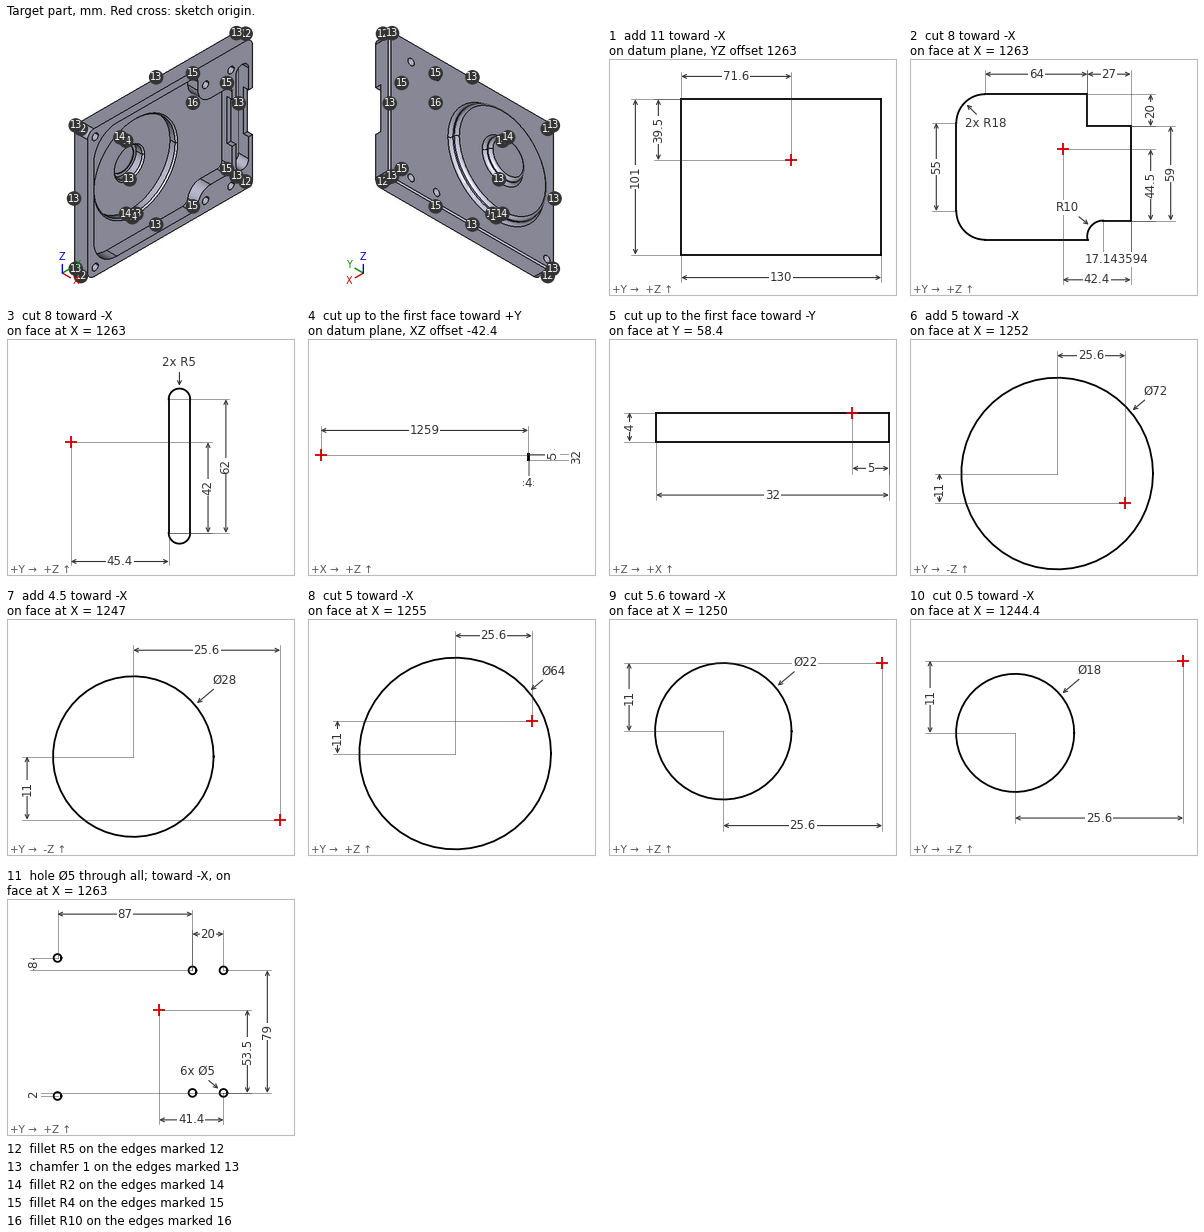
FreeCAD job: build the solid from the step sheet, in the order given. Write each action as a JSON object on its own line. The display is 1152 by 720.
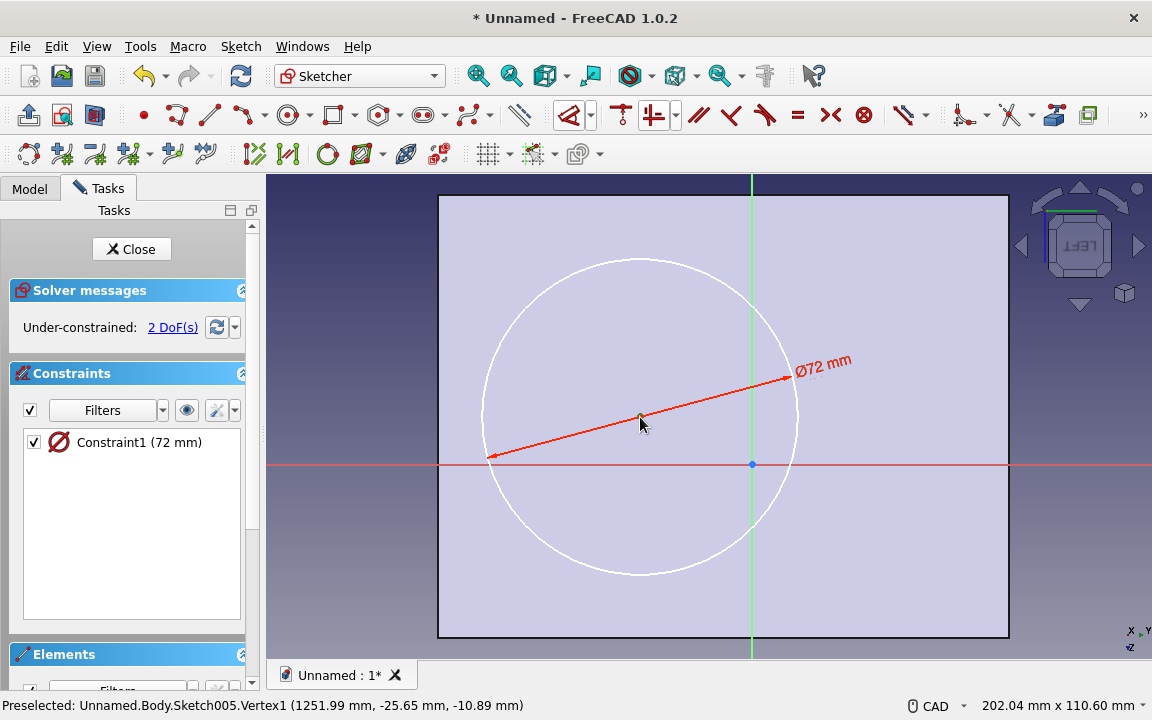
{"action": "left_click", "coordinate": [590, 116]}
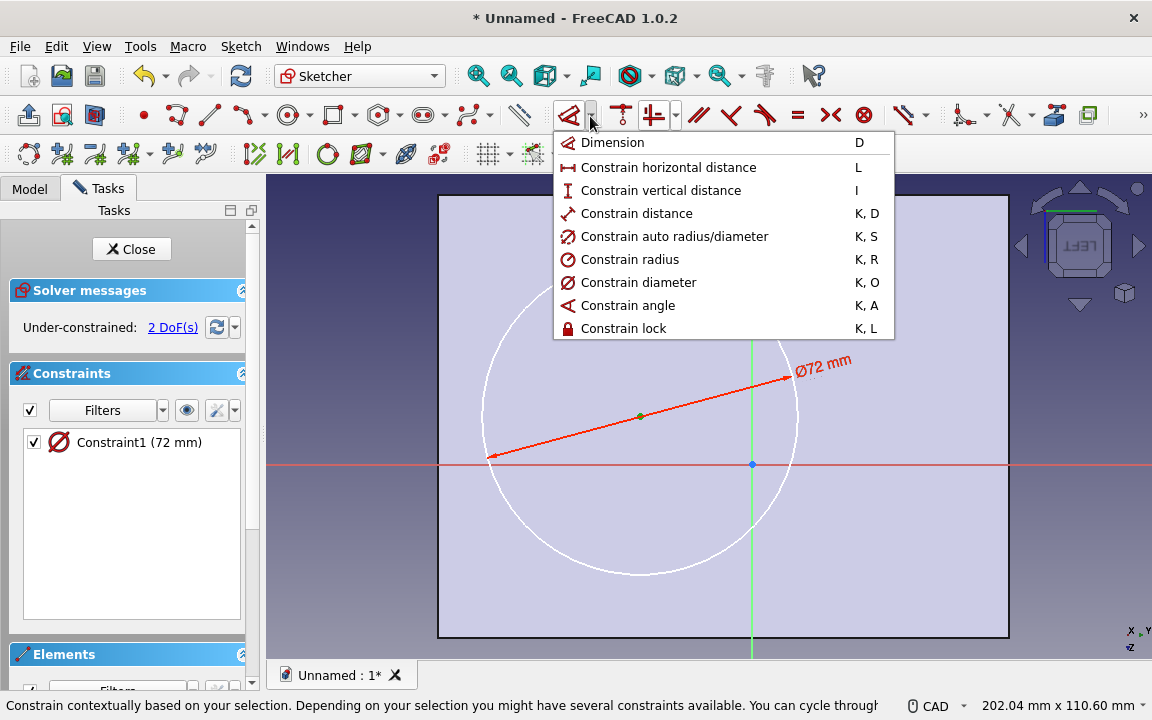
{"action": "left_click", "coordinate": [724, 190]}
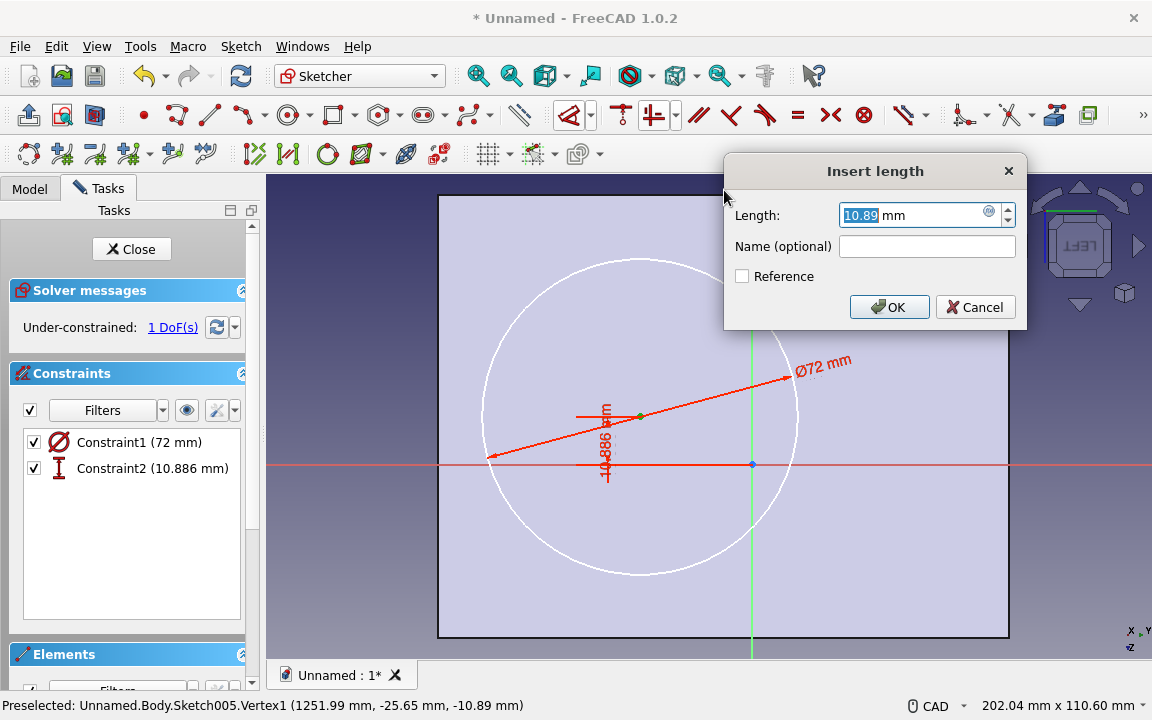
{"action": "type", "text": "11"}
{"action": "key", "text": "Return"}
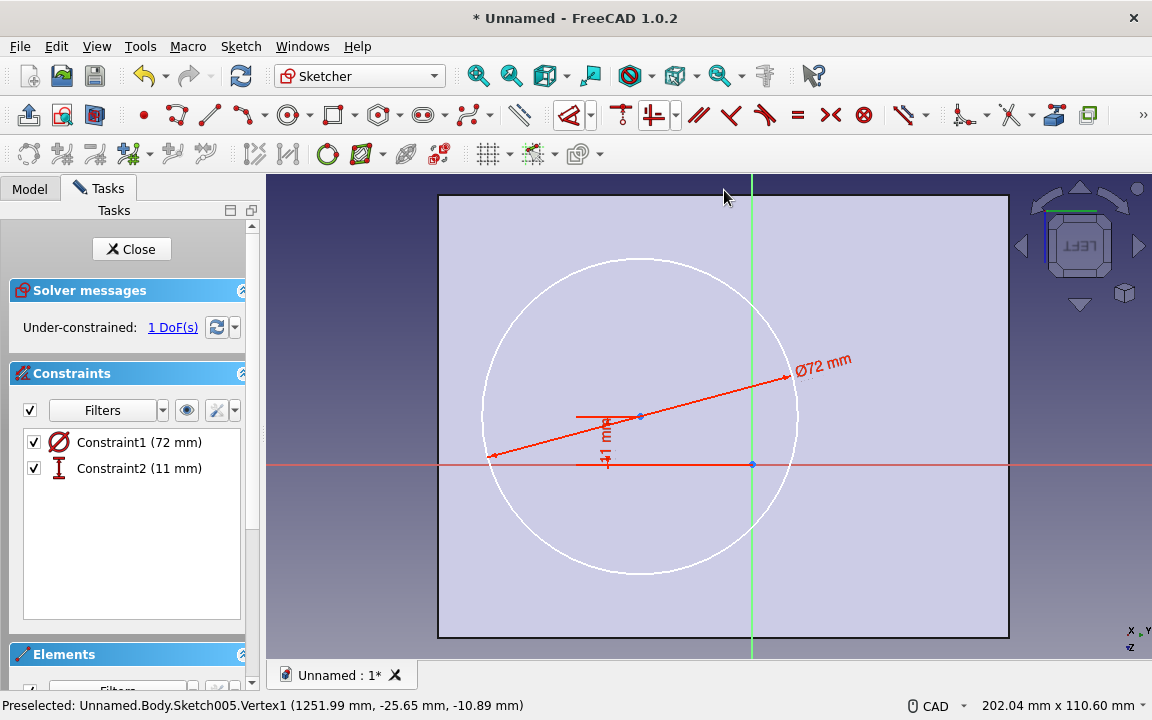
{"action": "left_click", "coordinate": [640, 416]}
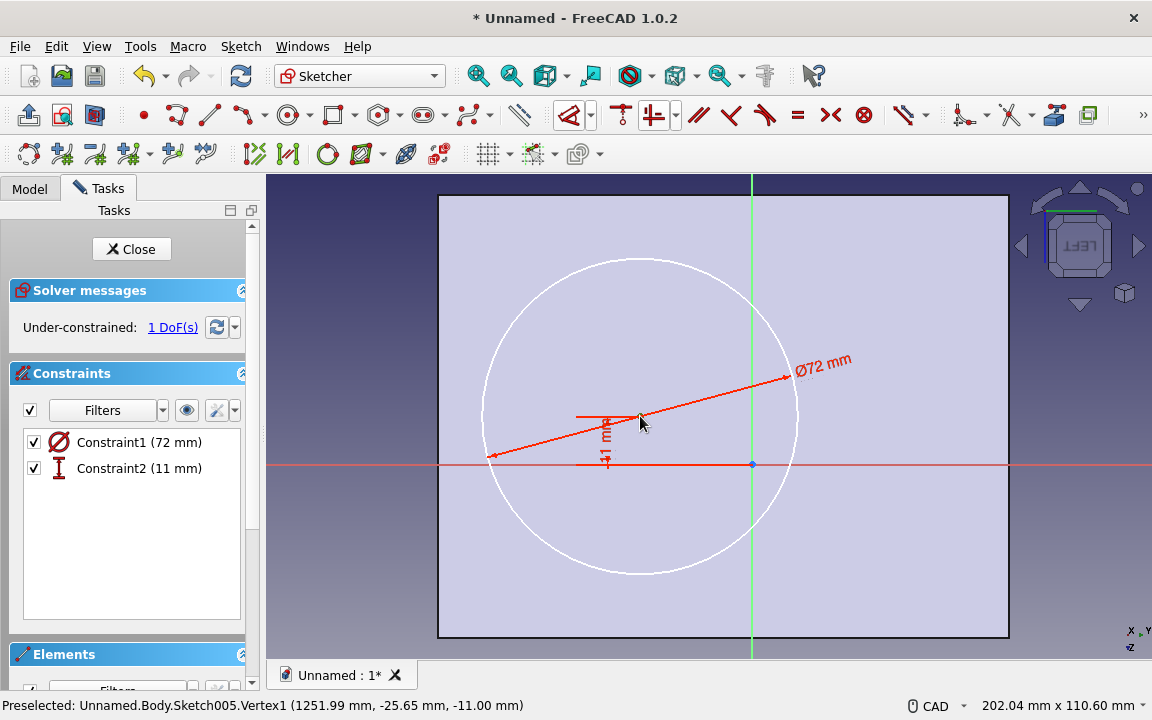
{"action": "left_click", "coordinate": [590, 116]}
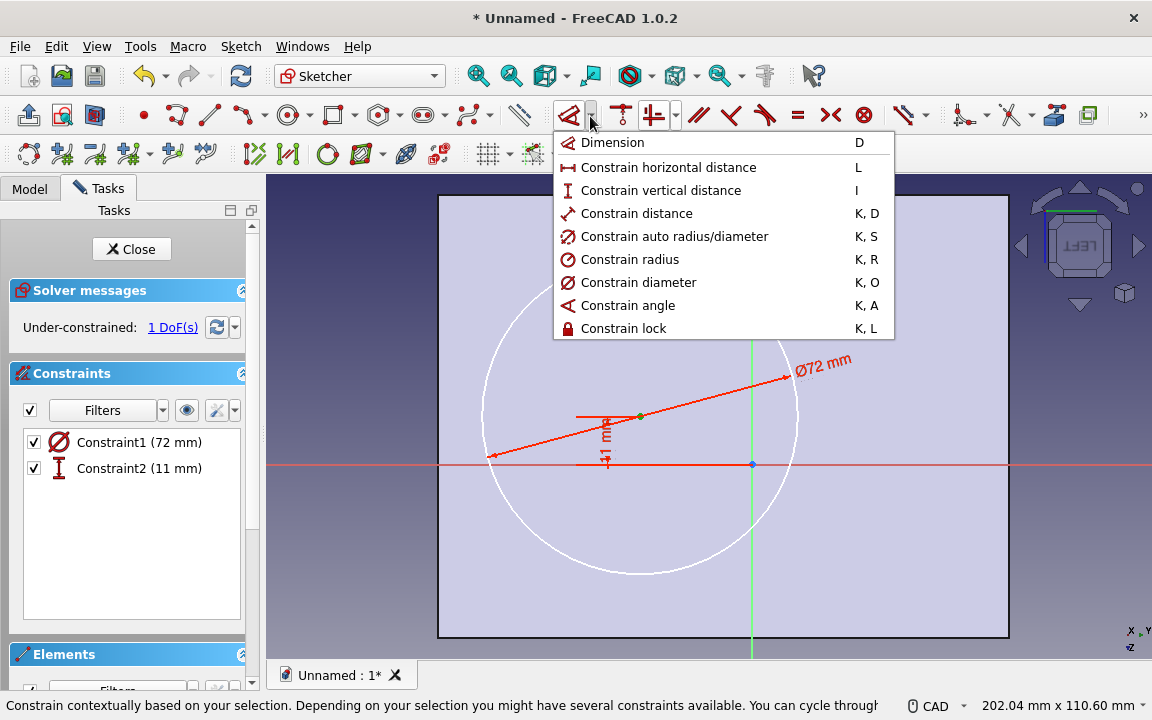
{"action": "left_click", "coordinate": [724, 168]}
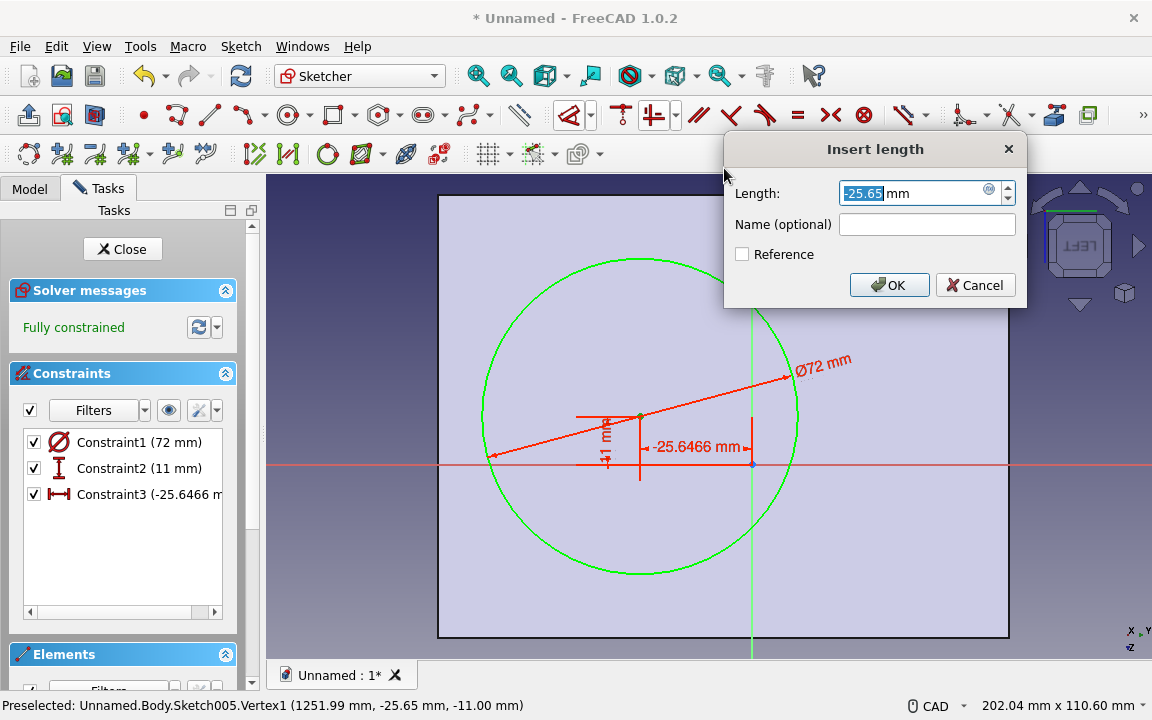
{"action": "type", "text": "-25.6"}
{"action": "key", "text": "Return"}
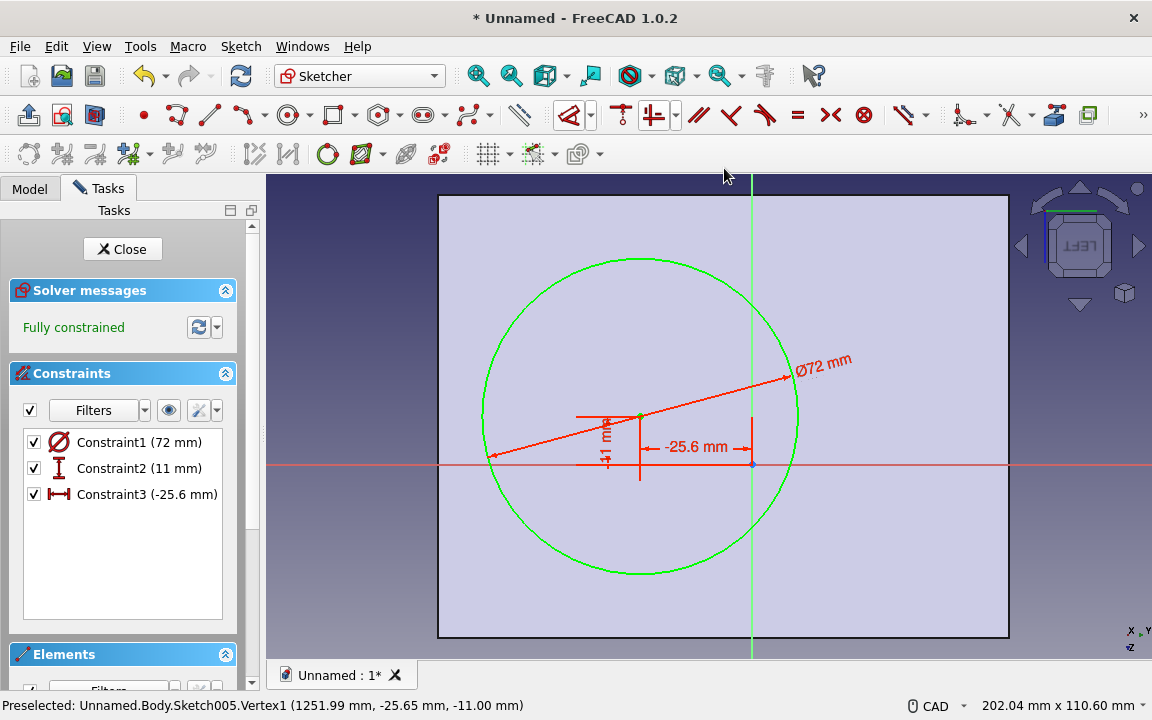
{"action": "left_click", "coordinate": [123, 249]}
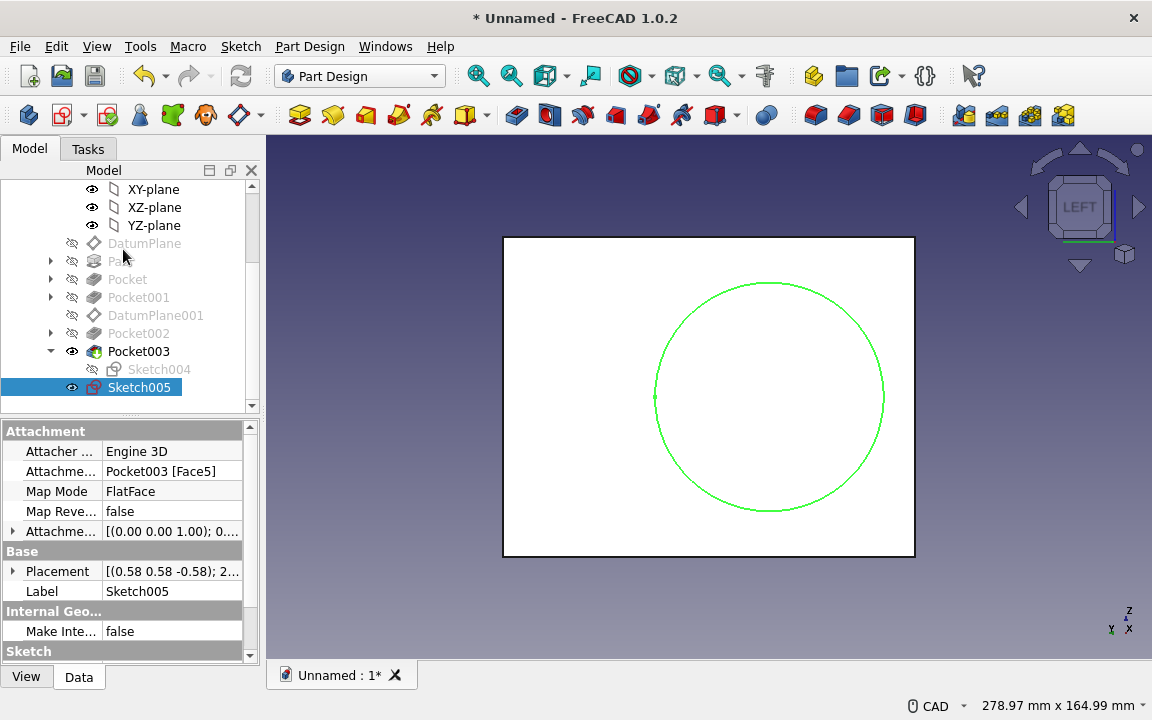
{"action": "left_click", "coordinate": [300, 116]}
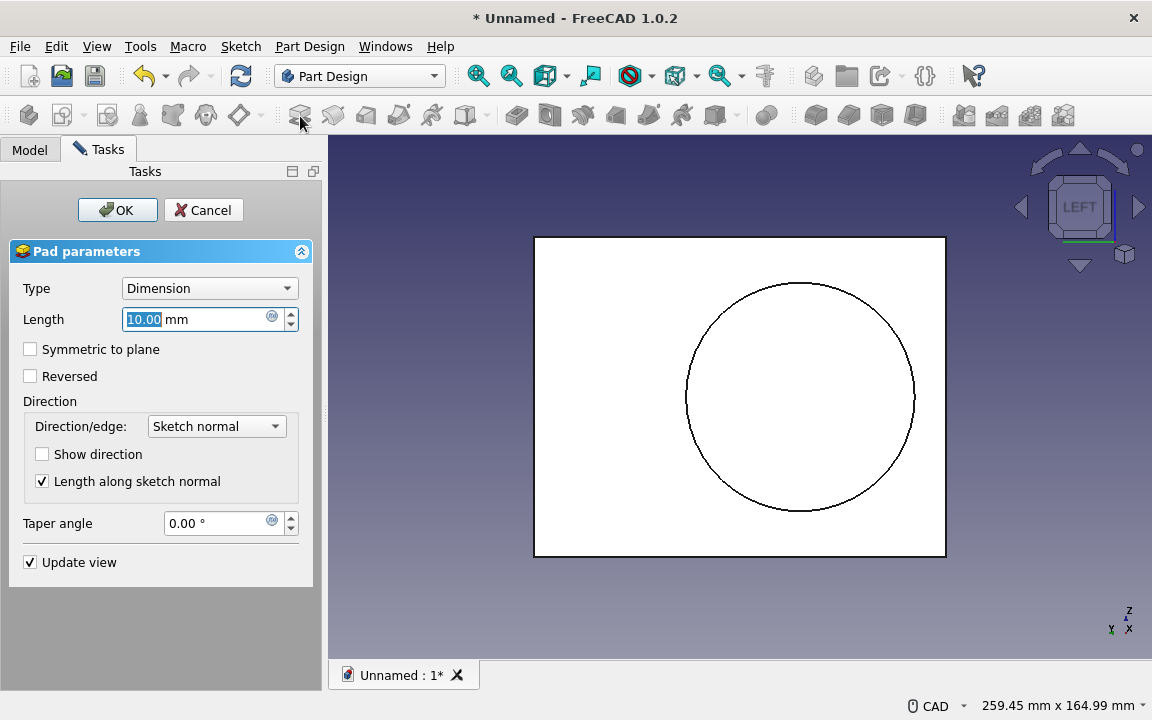
{"action": "type", "text": "5"}
{"action": "key", "text": "Tab"}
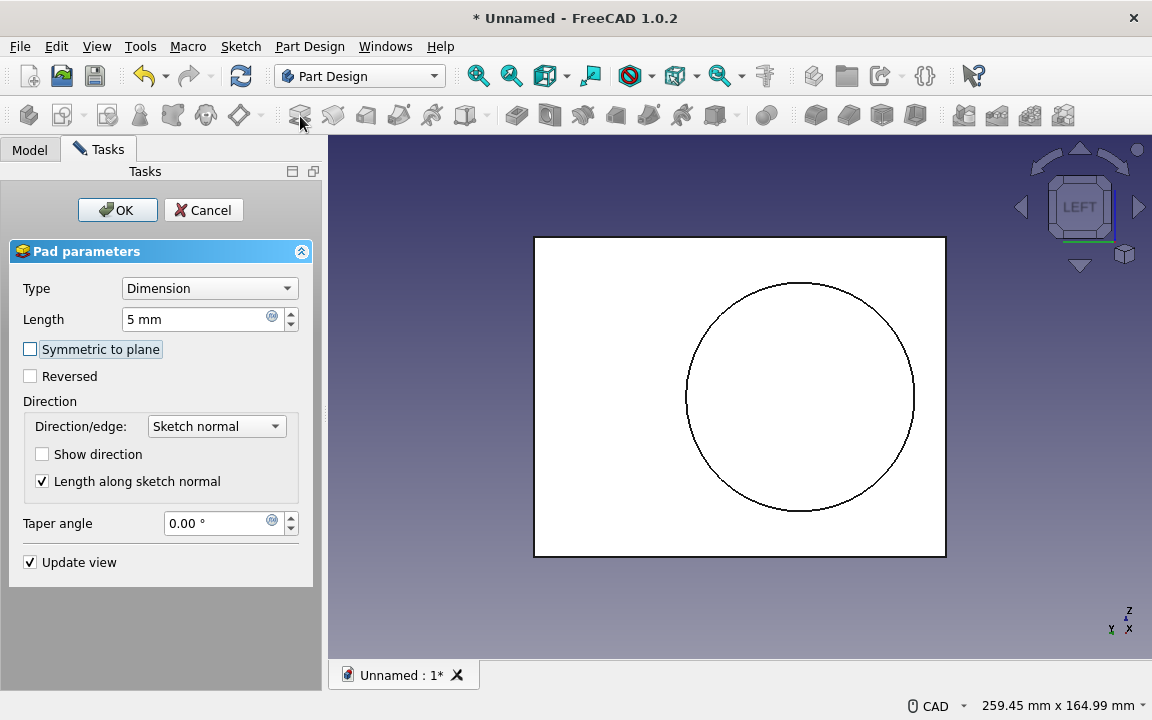
{"action": "left_click", "coordinate": [118, 210]}